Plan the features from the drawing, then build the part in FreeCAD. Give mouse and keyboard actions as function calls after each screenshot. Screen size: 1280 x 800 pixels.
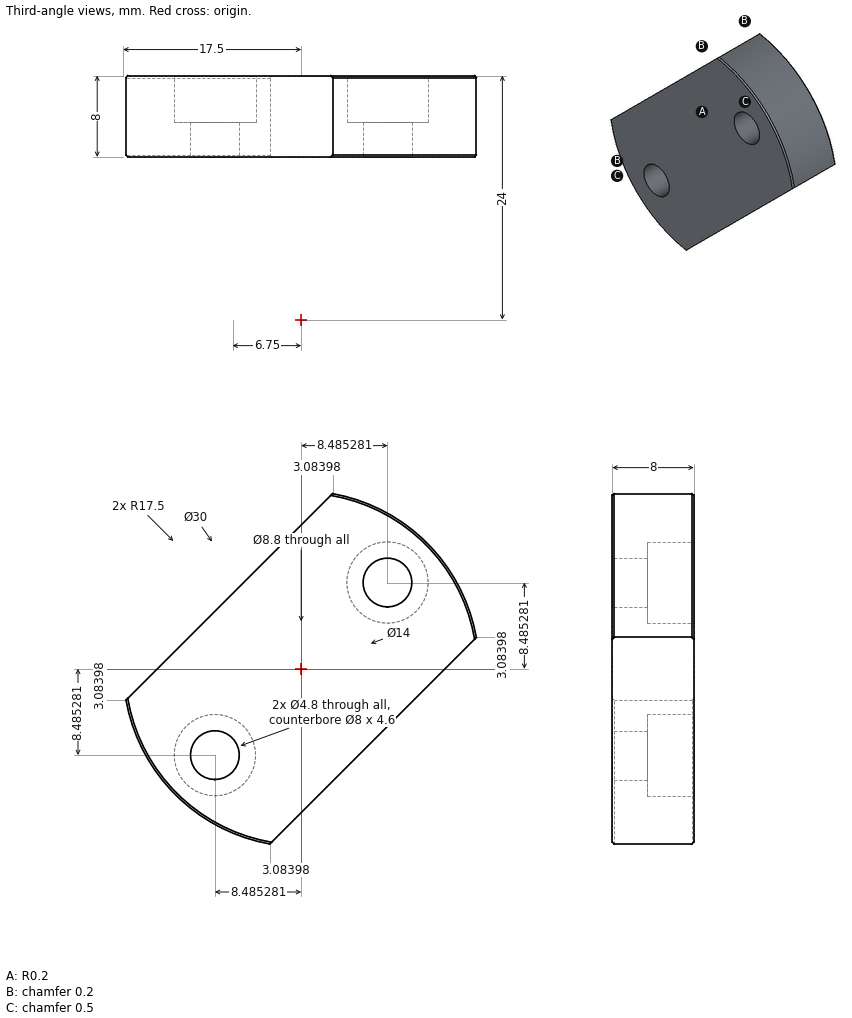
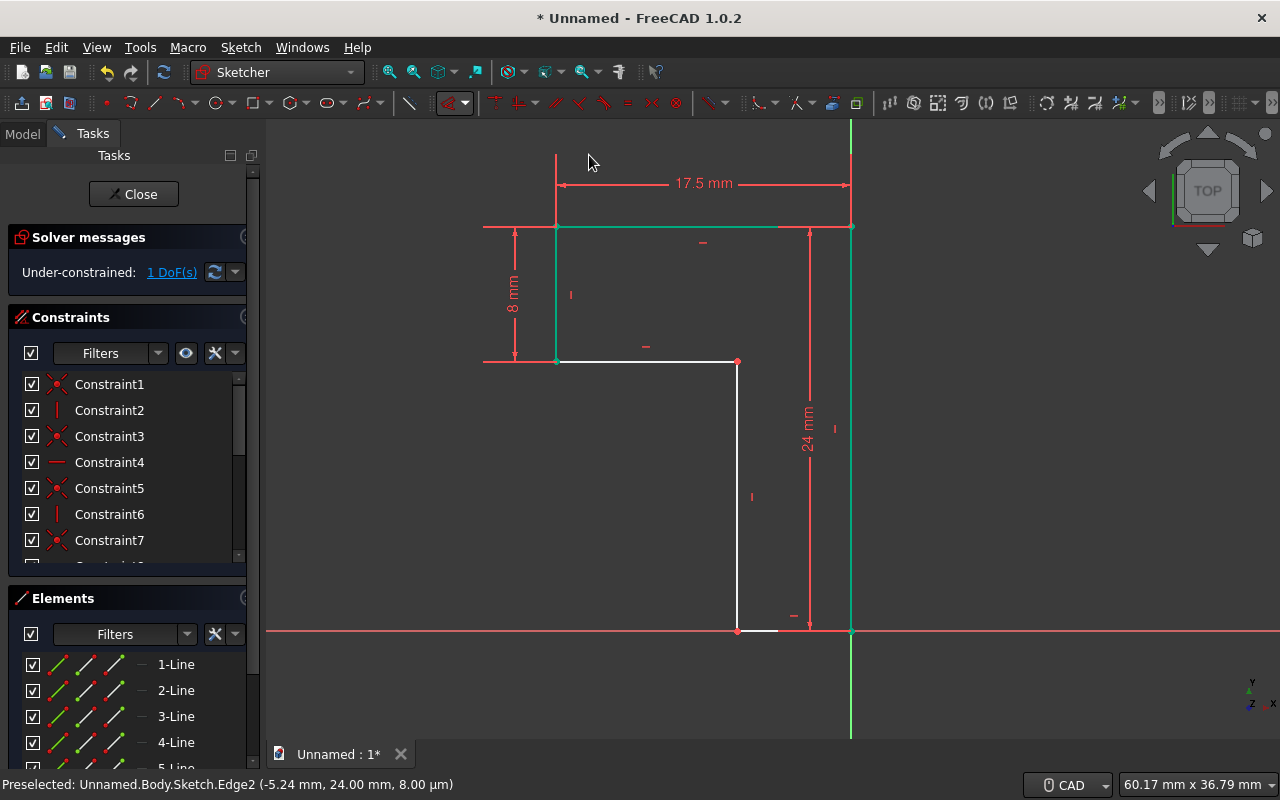
click(771, 631)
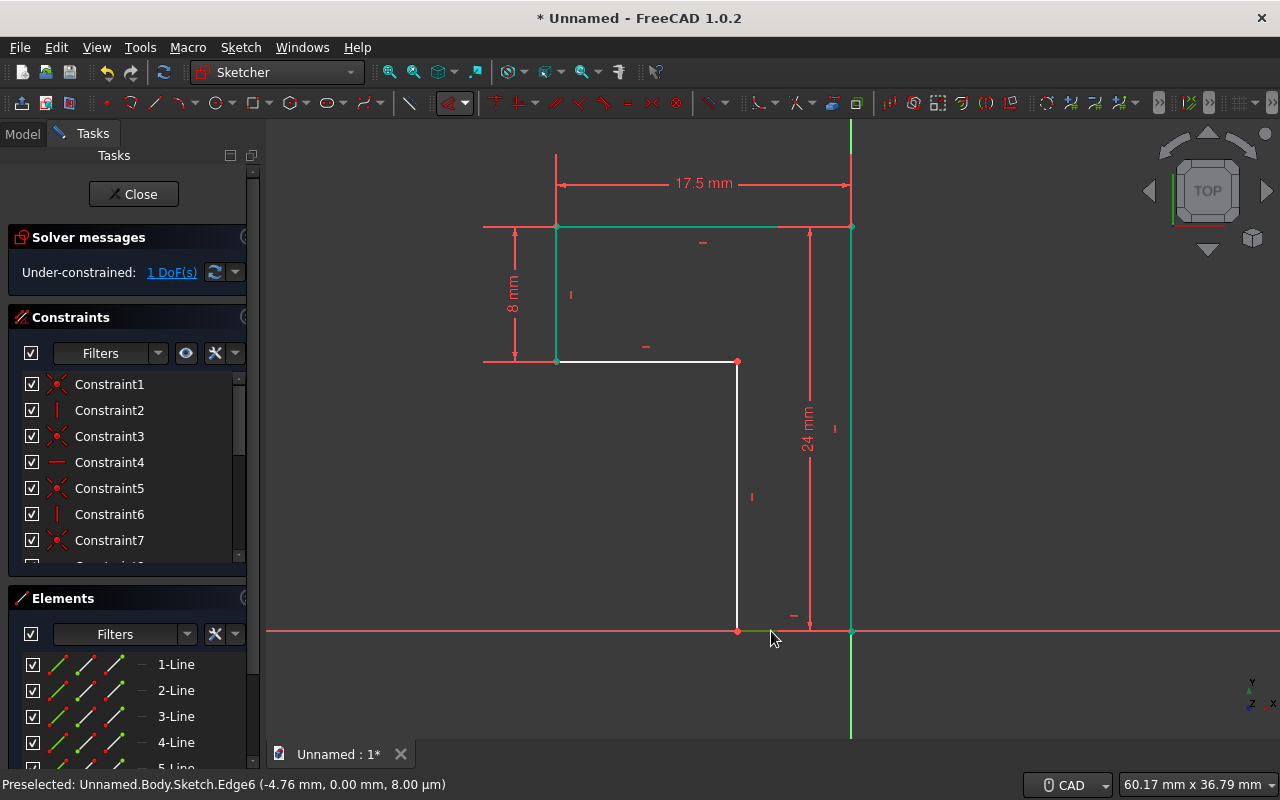
key(l)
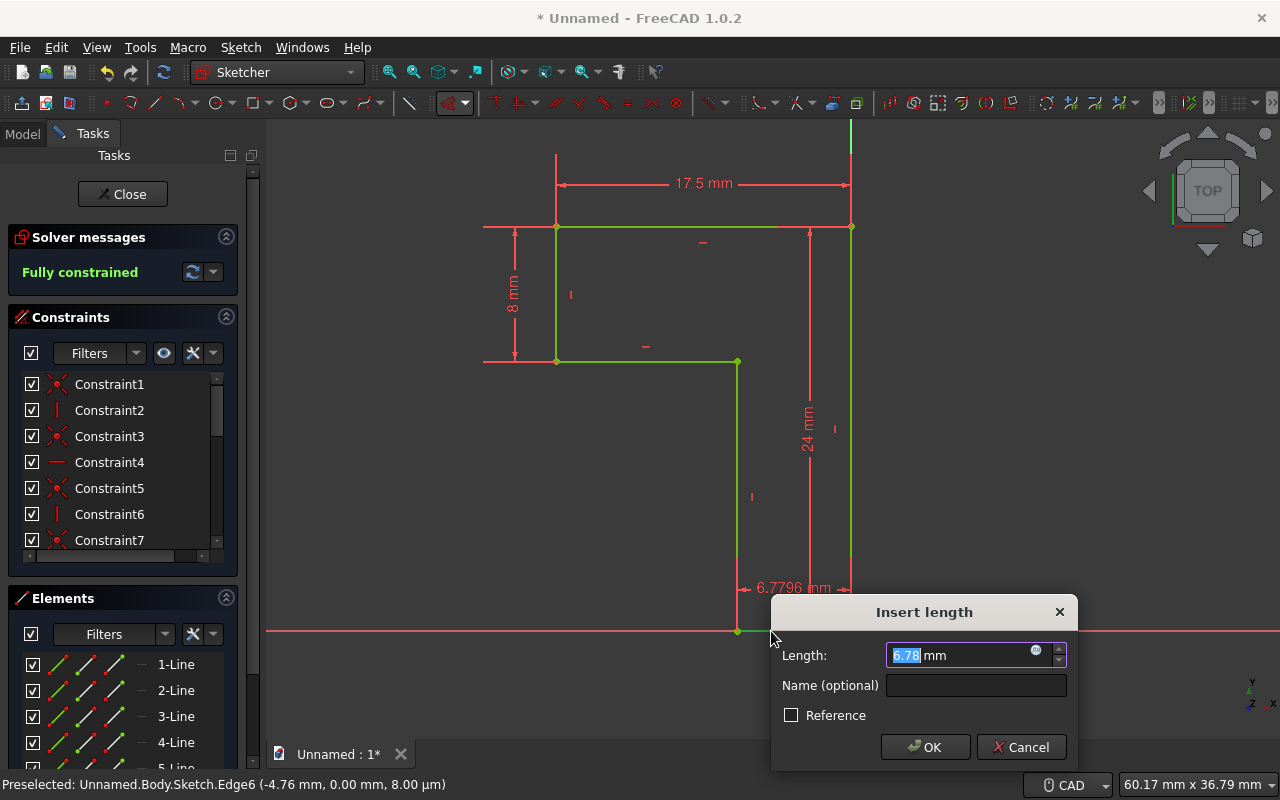
text(6.75)
key(Return)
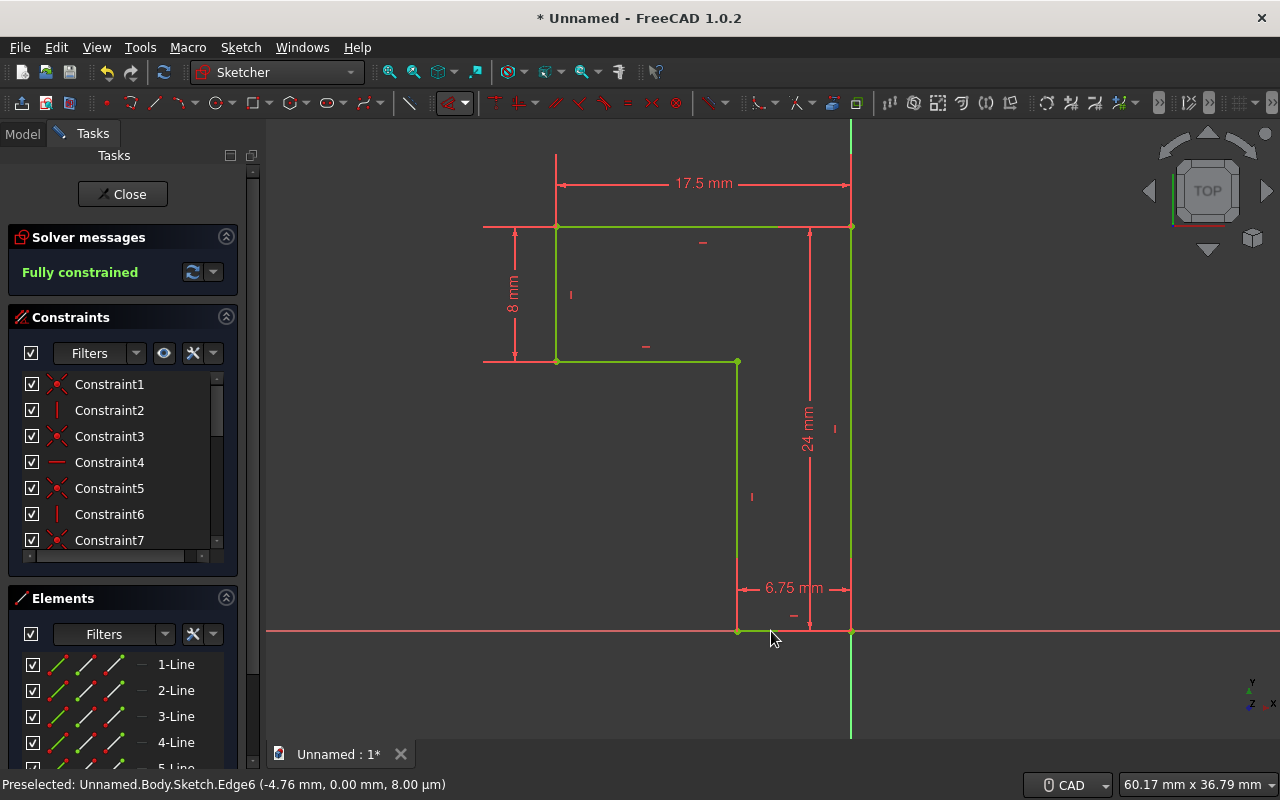
click(123, 194)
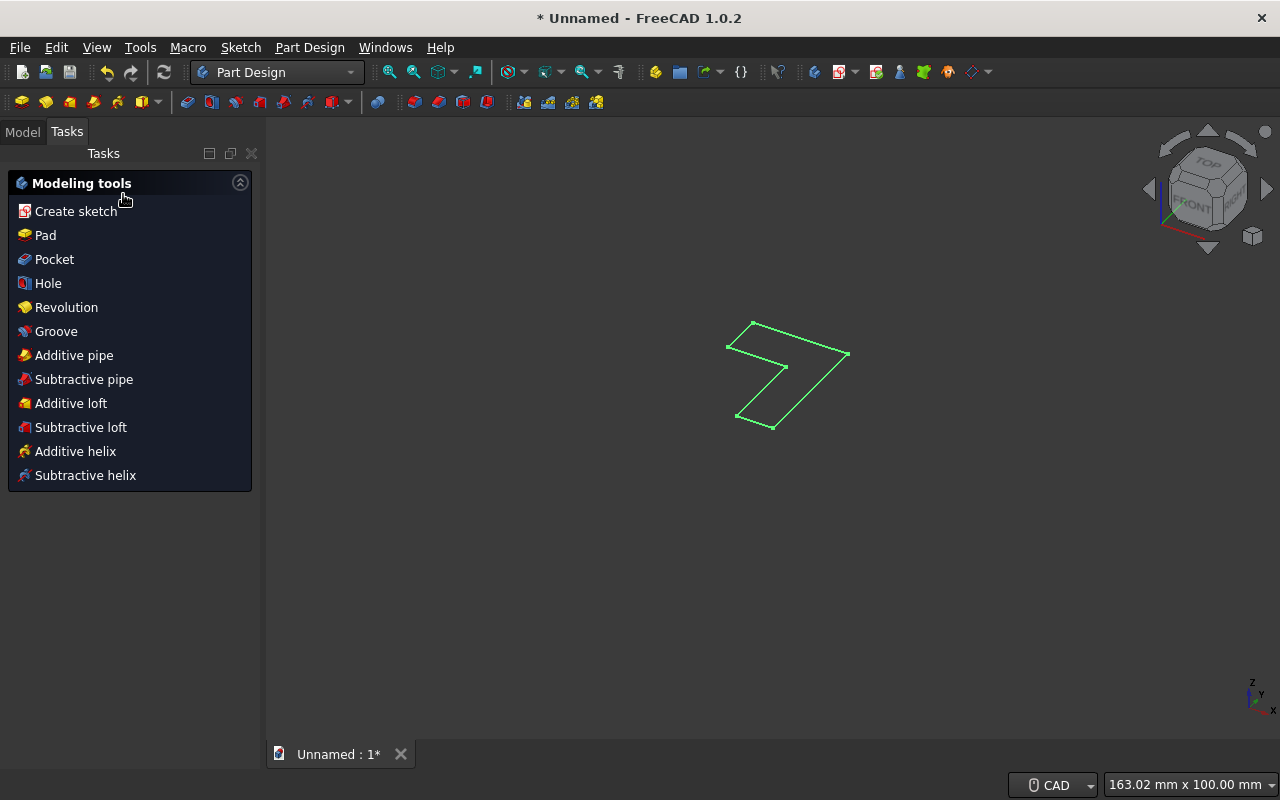
click(46, 102)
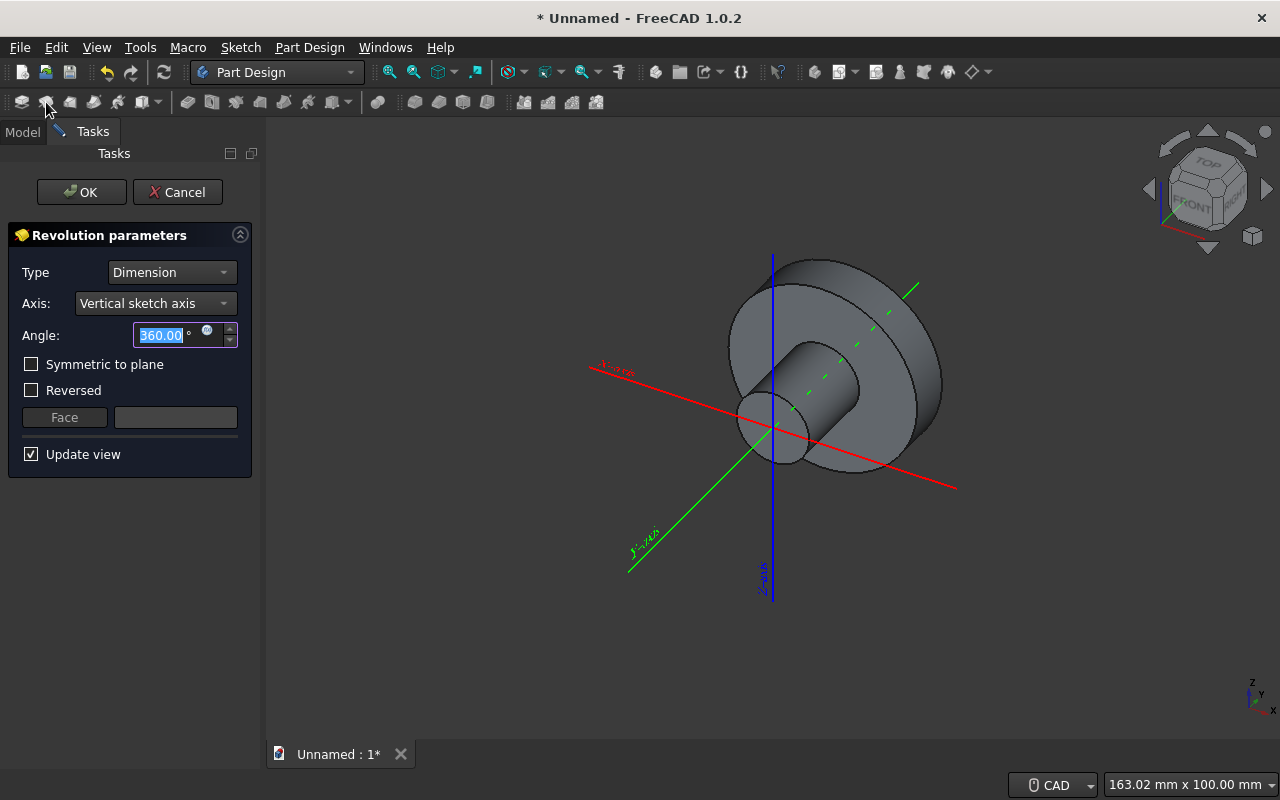
click(82, 192)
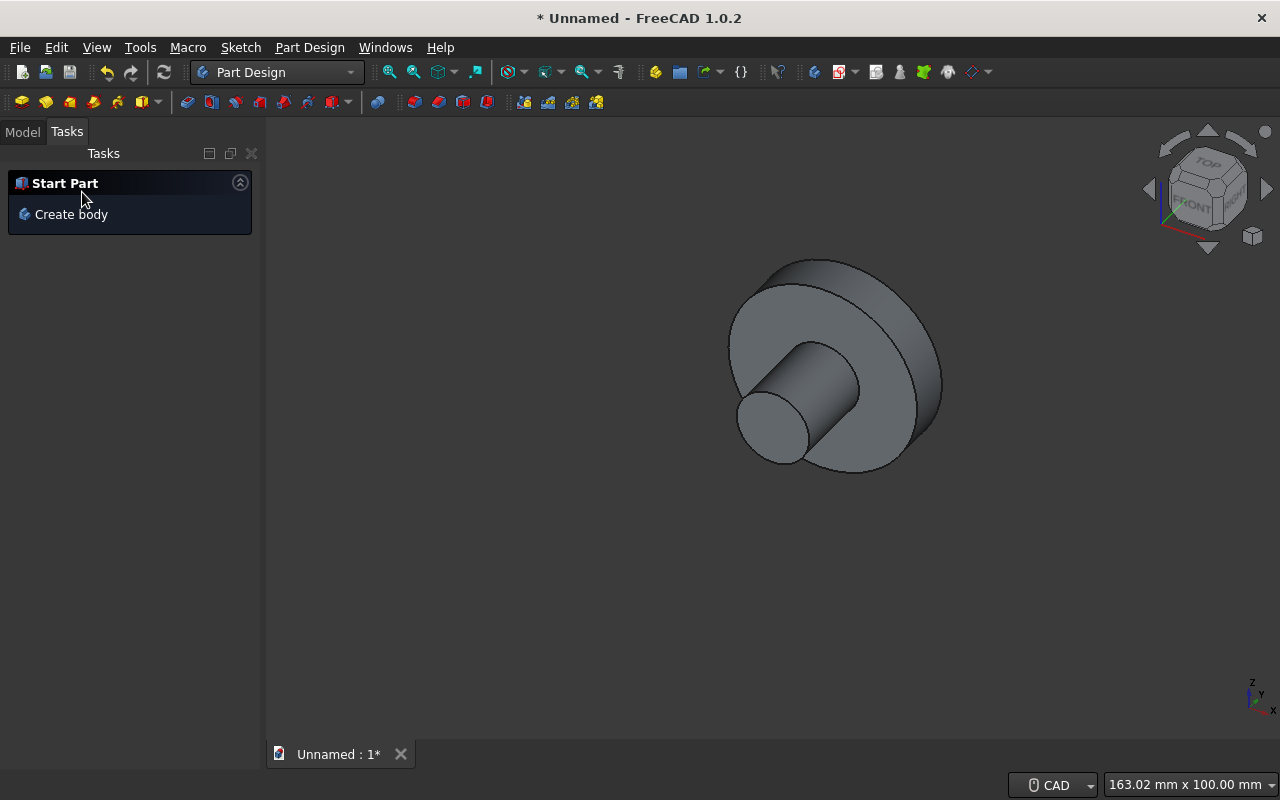
key(4)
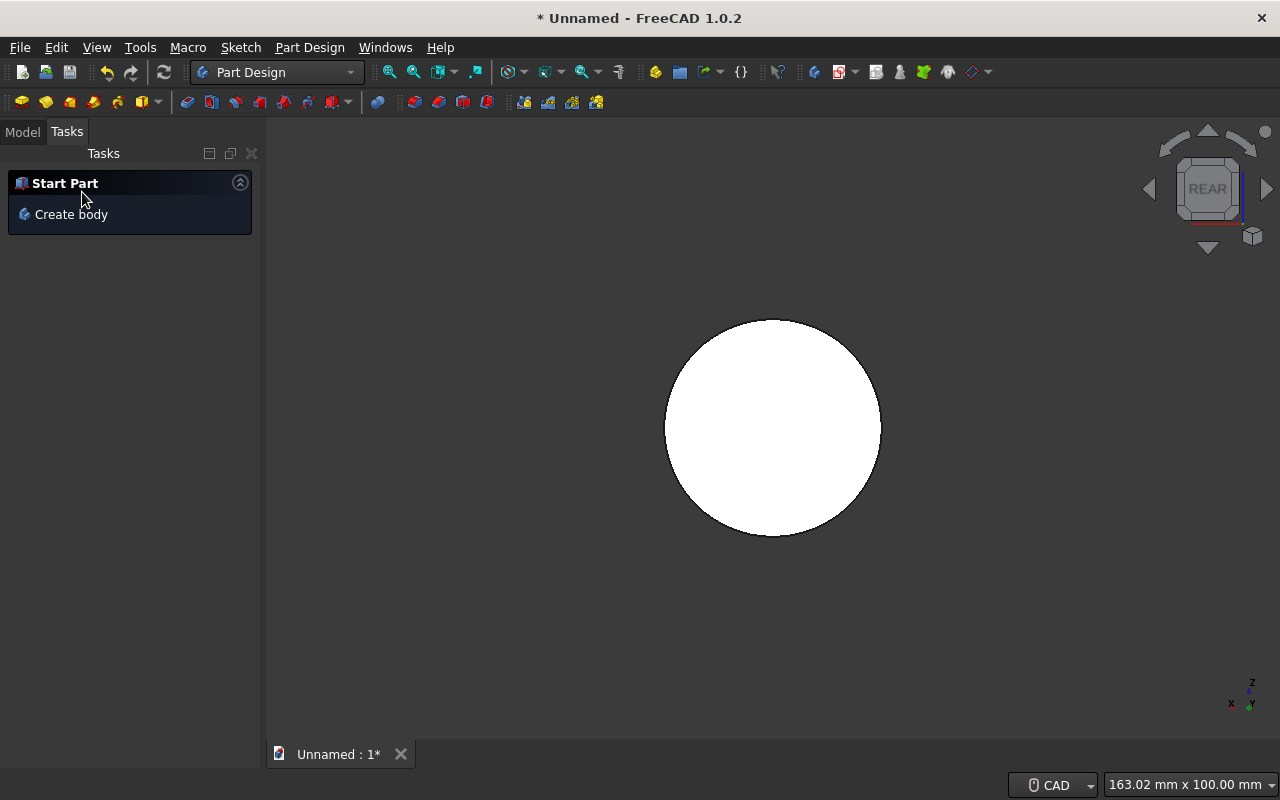
click(390, 72)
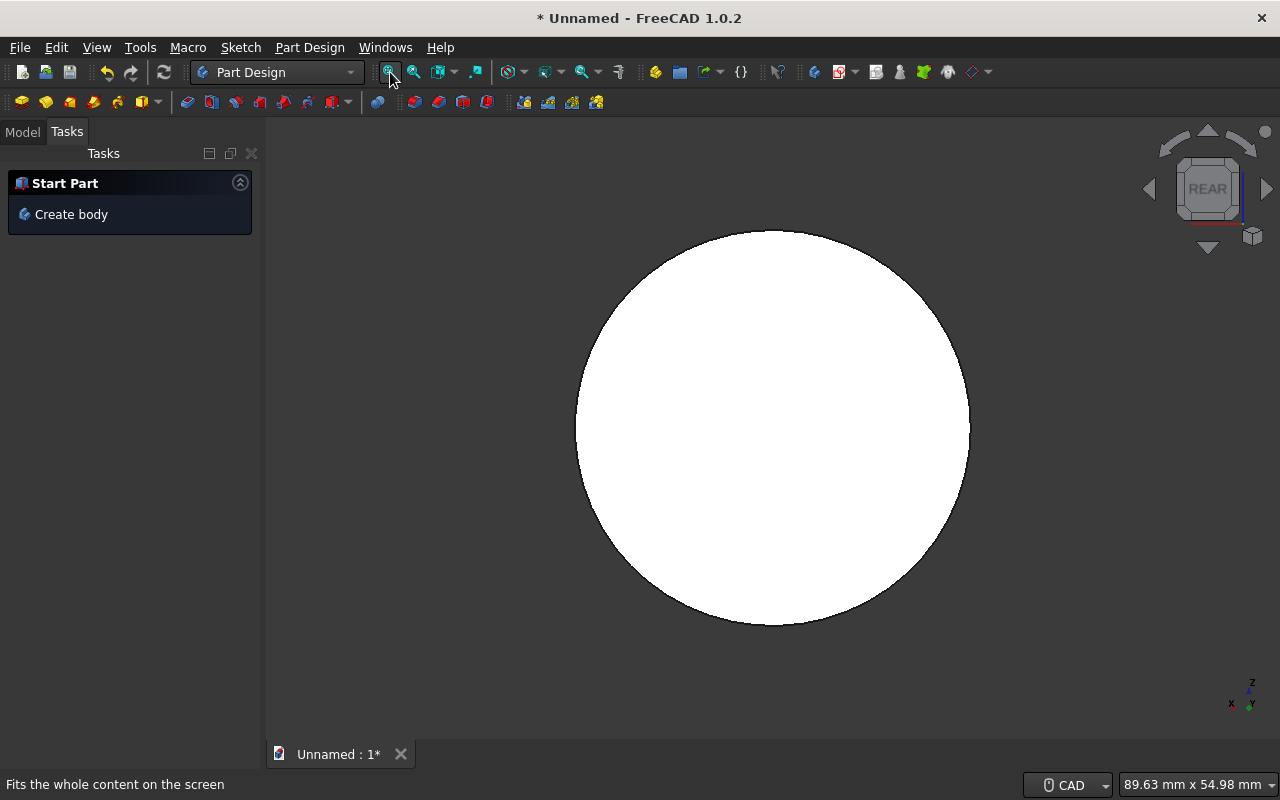
click(773, 427)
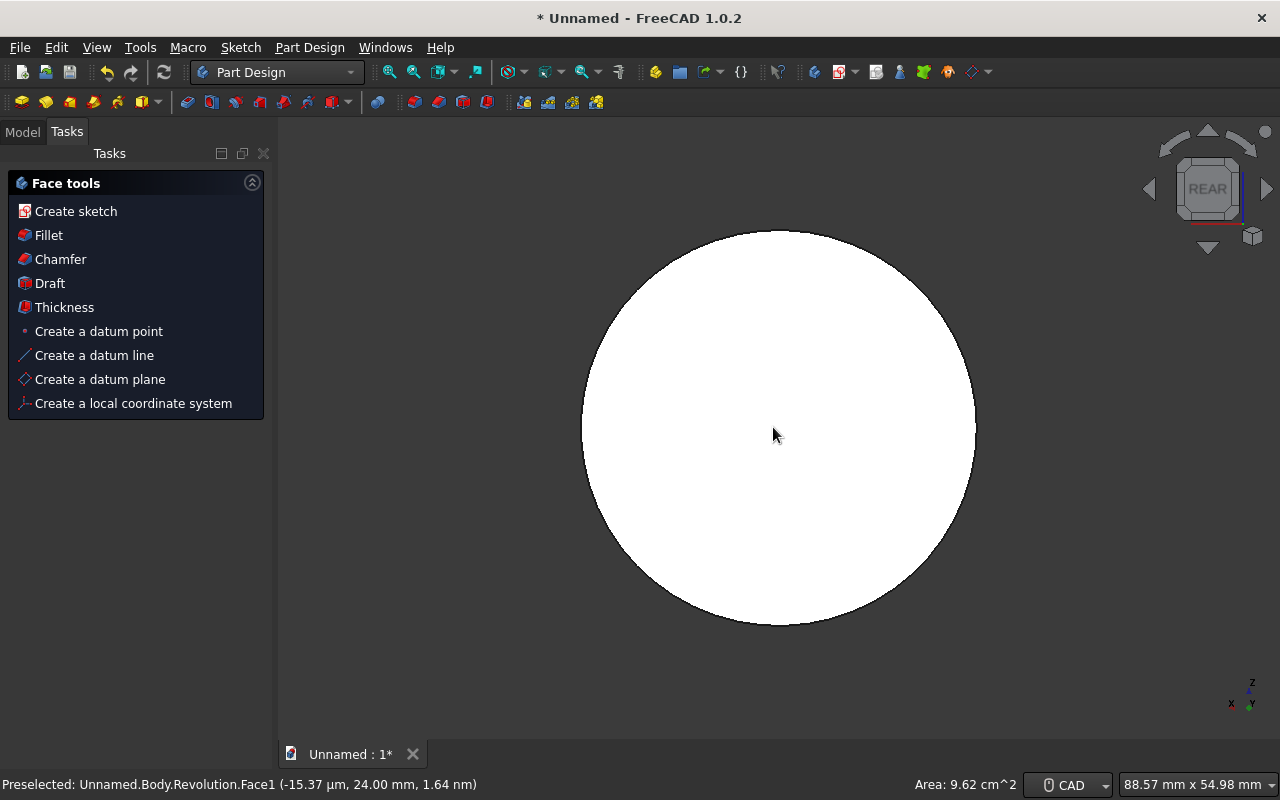
click(840, 72)